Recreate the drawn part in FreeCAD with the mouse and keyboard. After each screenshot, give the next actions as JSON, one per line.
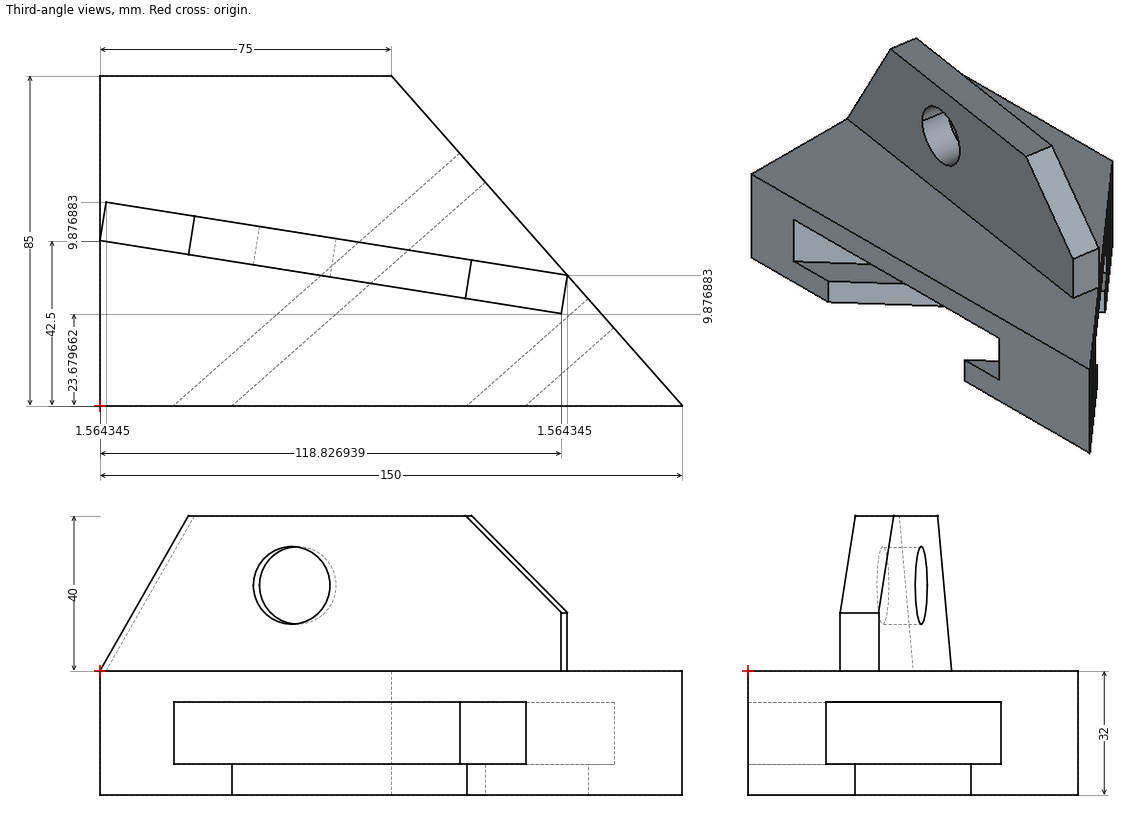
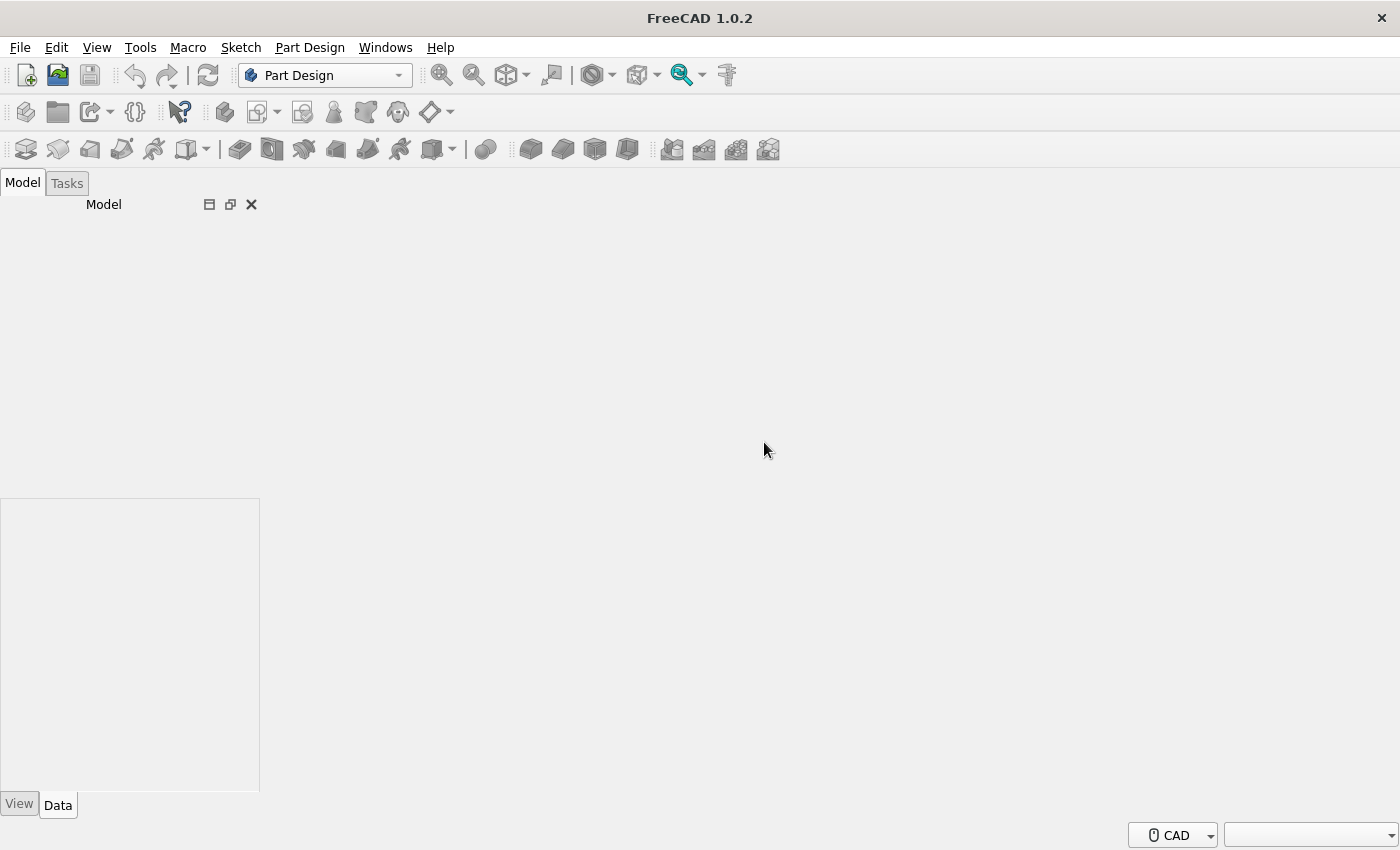
{"action": "key", "text": "ctrl+n"}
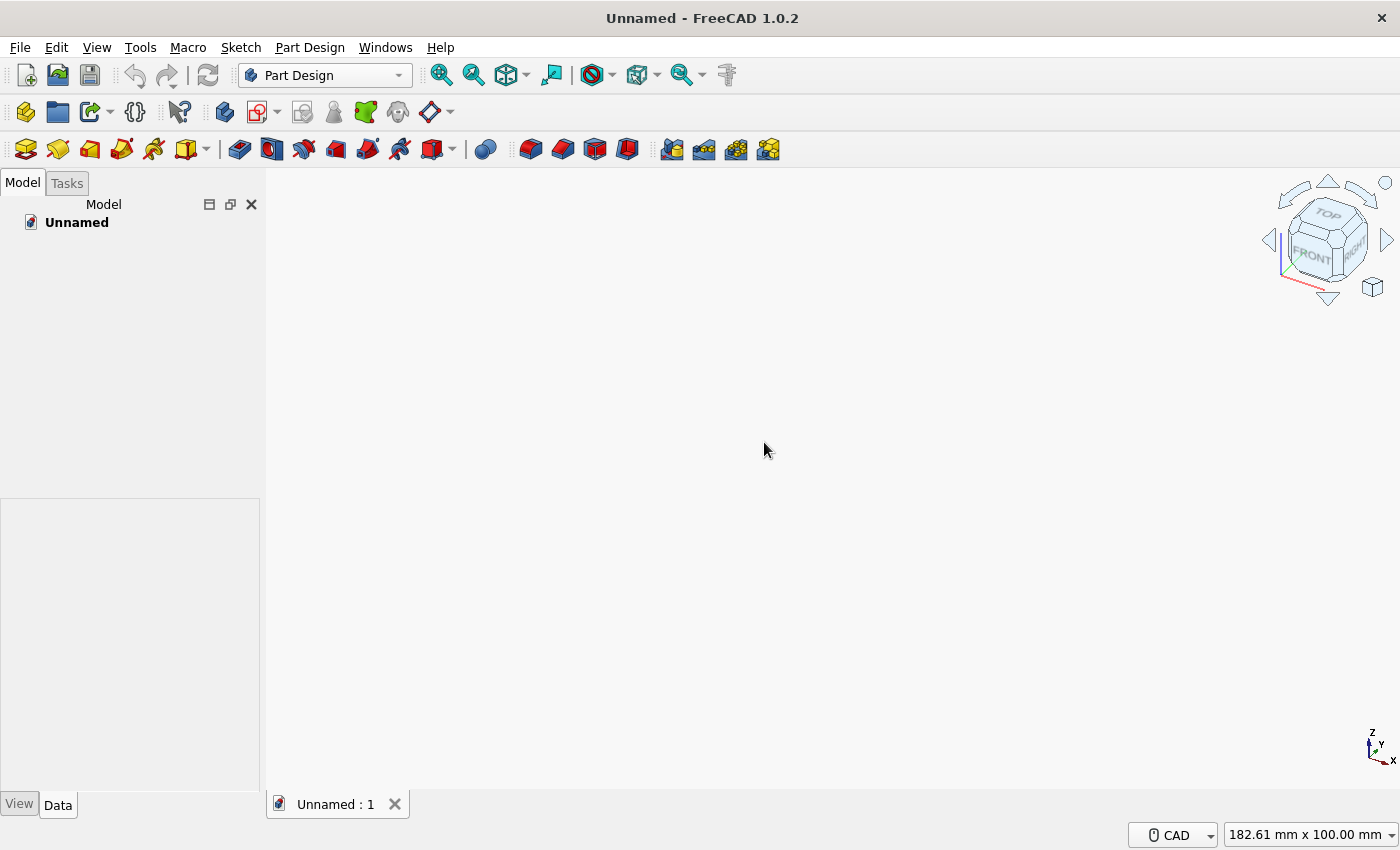
{"action": "left_click", "coordinate": [258, 112]}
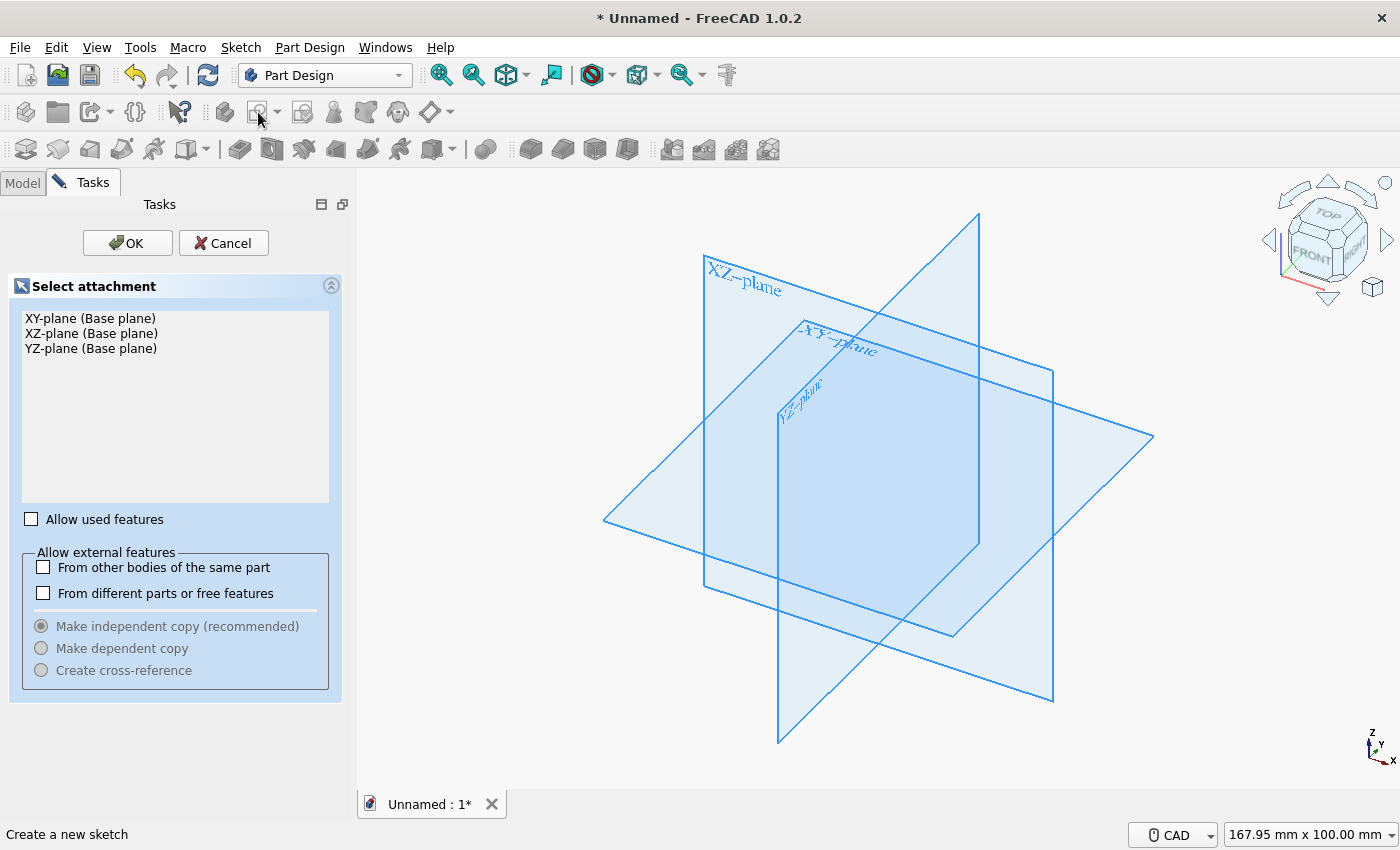
{"action": "left_click", "coordinate": [82, 318]}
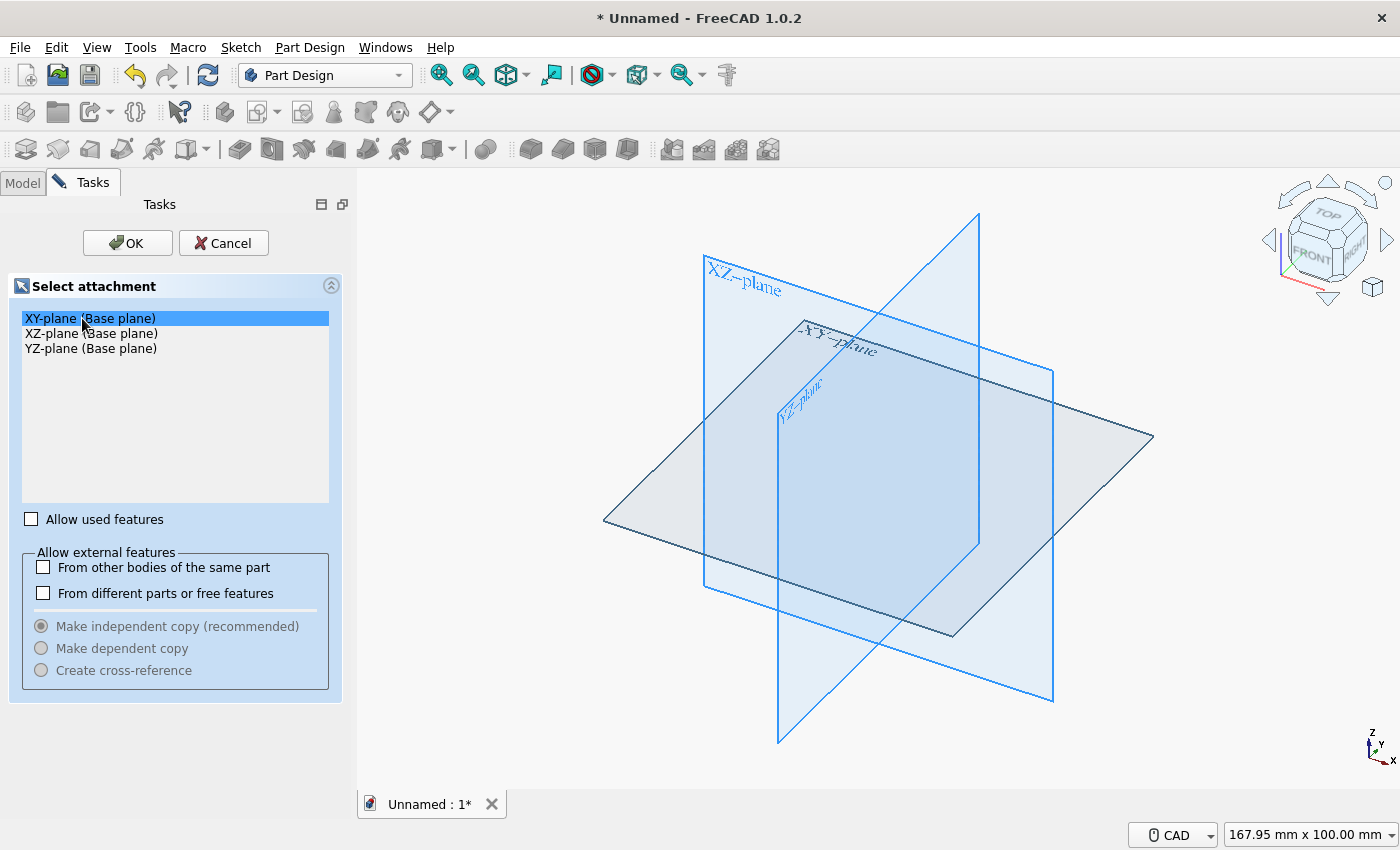
{"action": "left_click", "coordinate": [128, 243]}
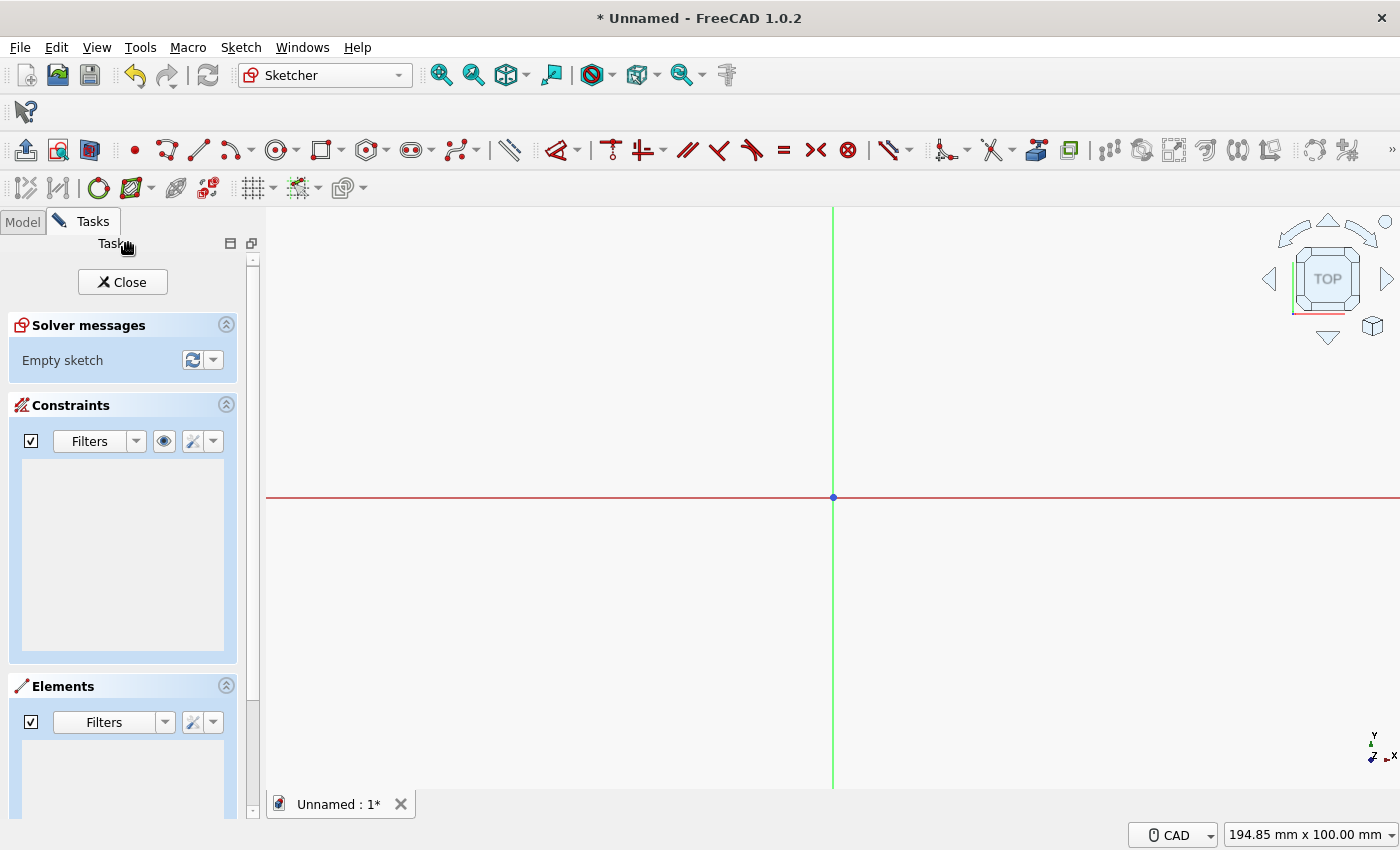
{"action": "scroll", "coordinate": [294, 761], "scroll_direction": "down", "scroll_amount": 3}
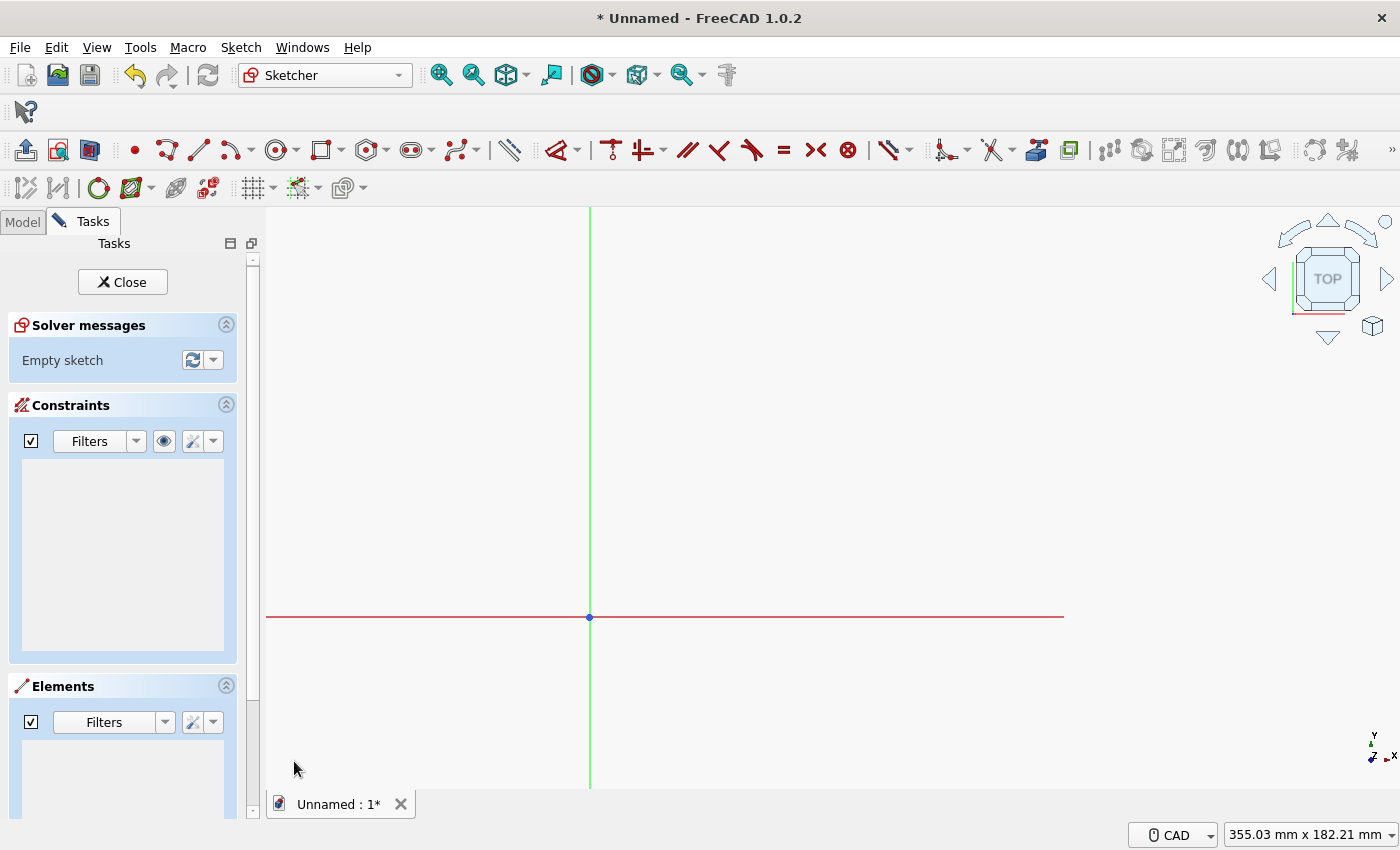
{"action": "scroll", "coordinate": [961, 447], "scroll_direction": "up", "scroll_amount": 2}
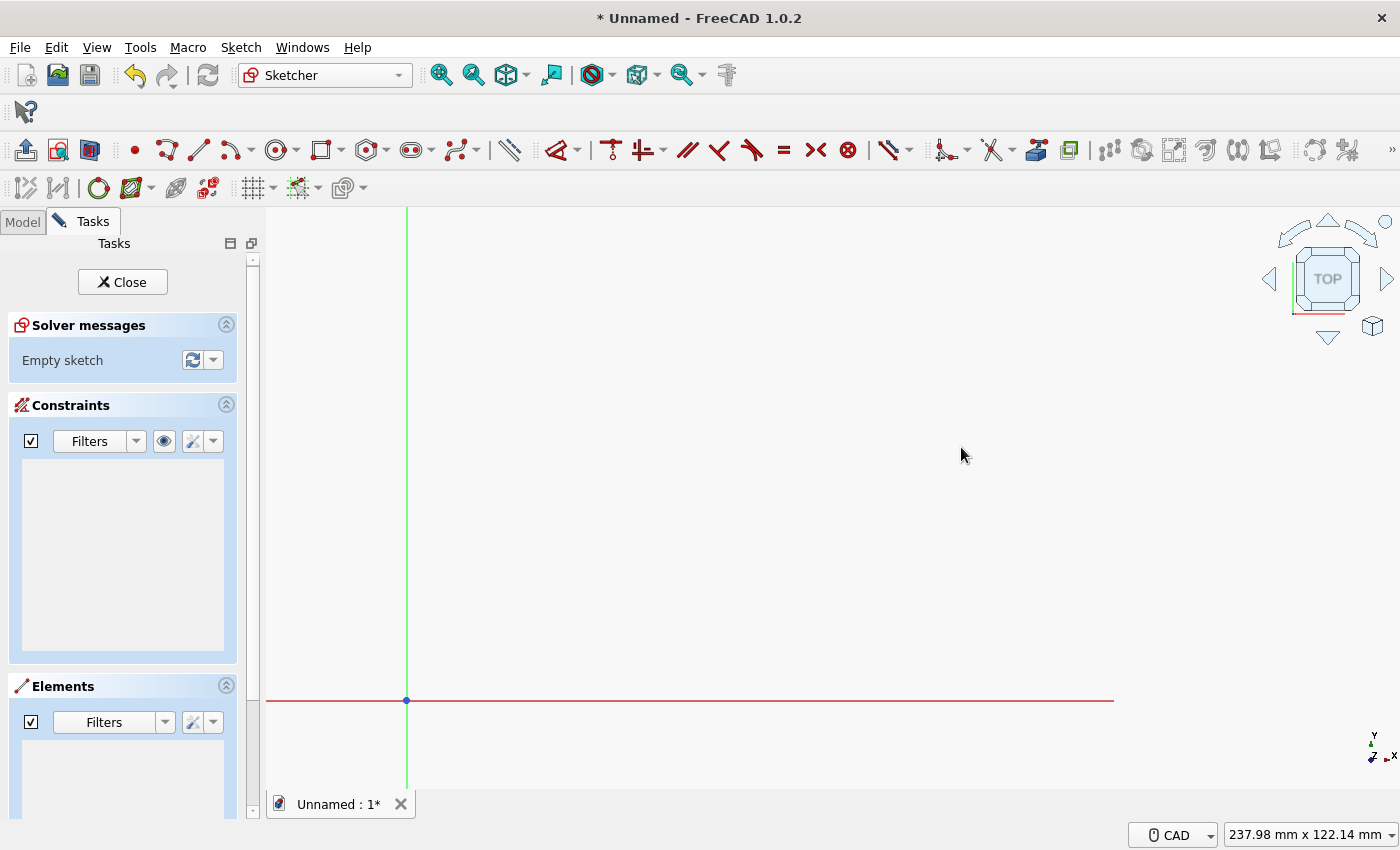
{"action": "key", "text": "g m"}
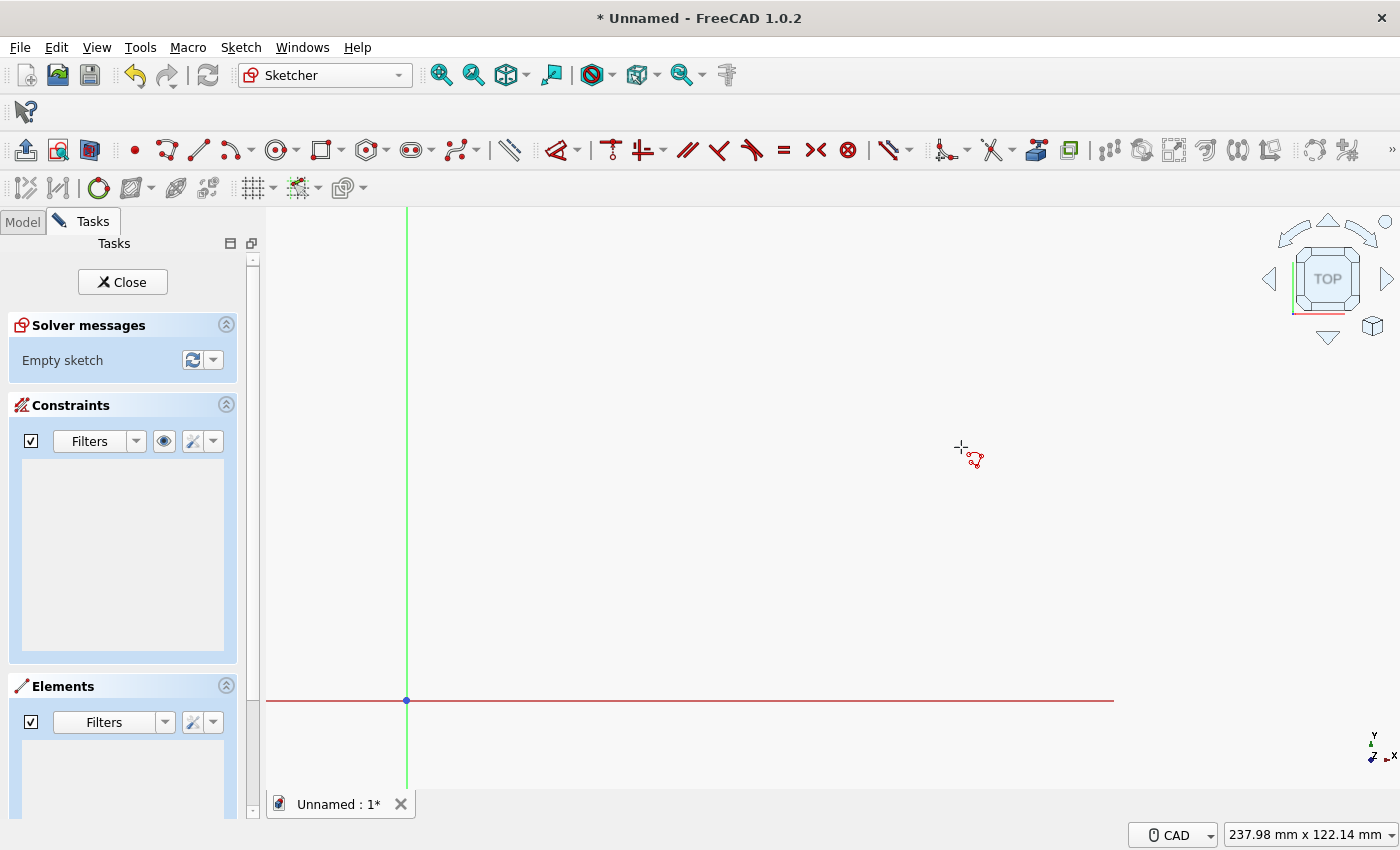
{"action": "left_click", "coordinate": [407, 701]}
{"action": "left_click", "coordinate": [1122, 692]}
{"action": "left_click", "coordinate": [764, 296]}
{"action": "left_click", "coordinate": [416, 296]}
{"action": "left_click", "coordinate": [407, 701]}
{"action": "key", "text": "Escape"}
{"action": "key", "text": "Escape"}